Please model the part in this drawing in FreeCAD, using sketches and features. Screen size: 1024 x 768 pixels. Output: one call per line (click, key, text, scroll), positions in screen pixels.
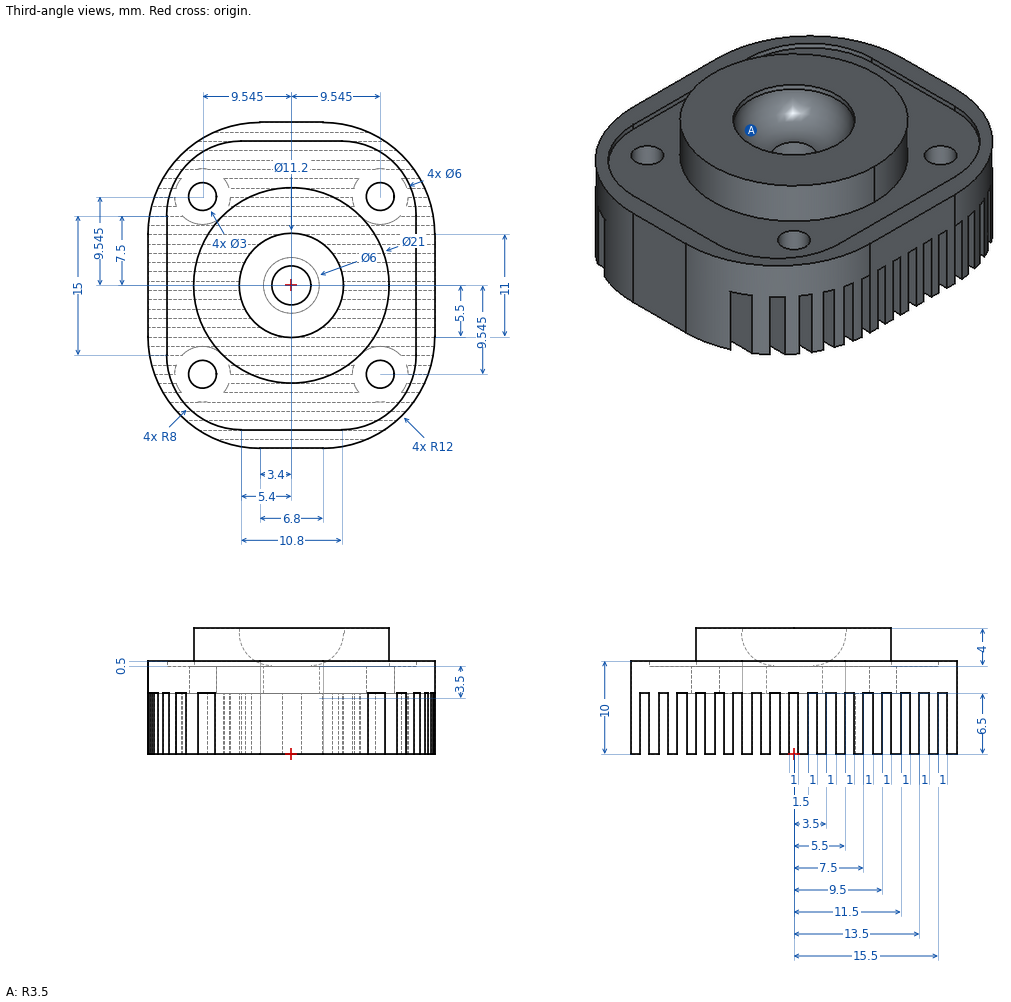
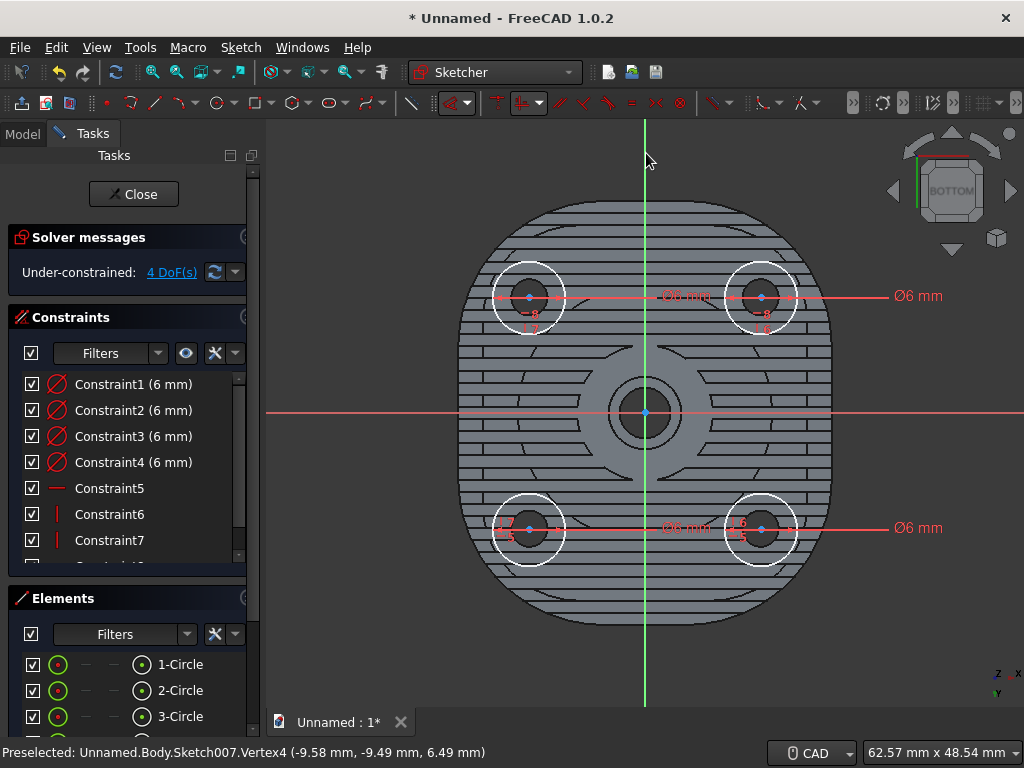
click(761, 530)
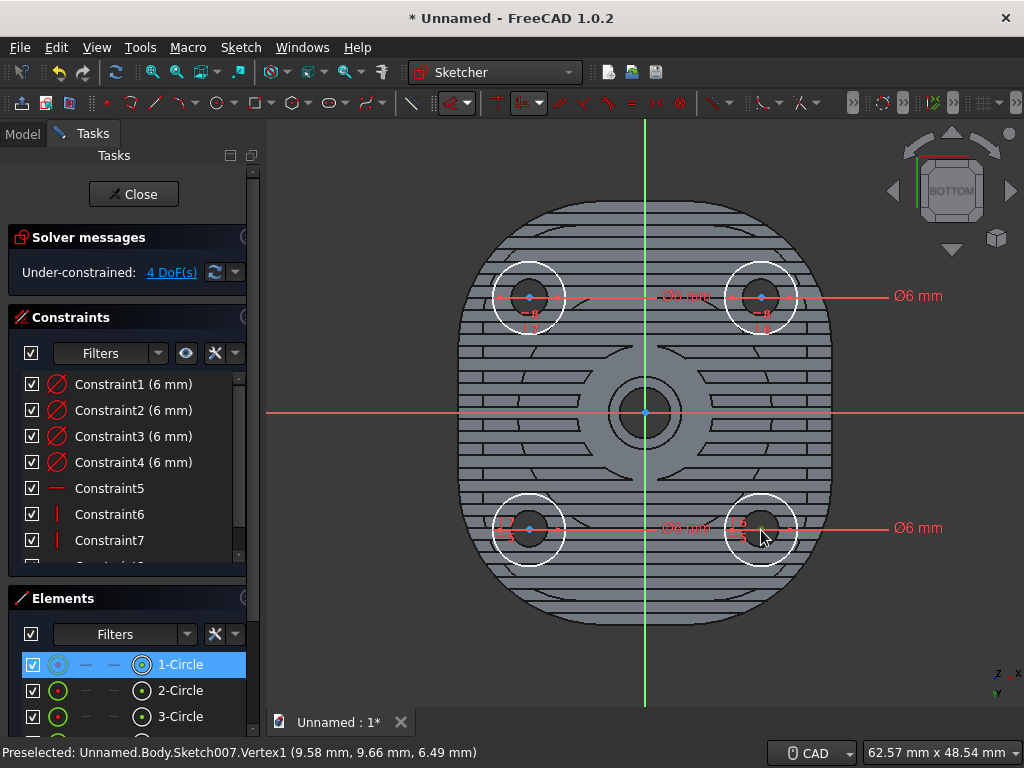
key(l)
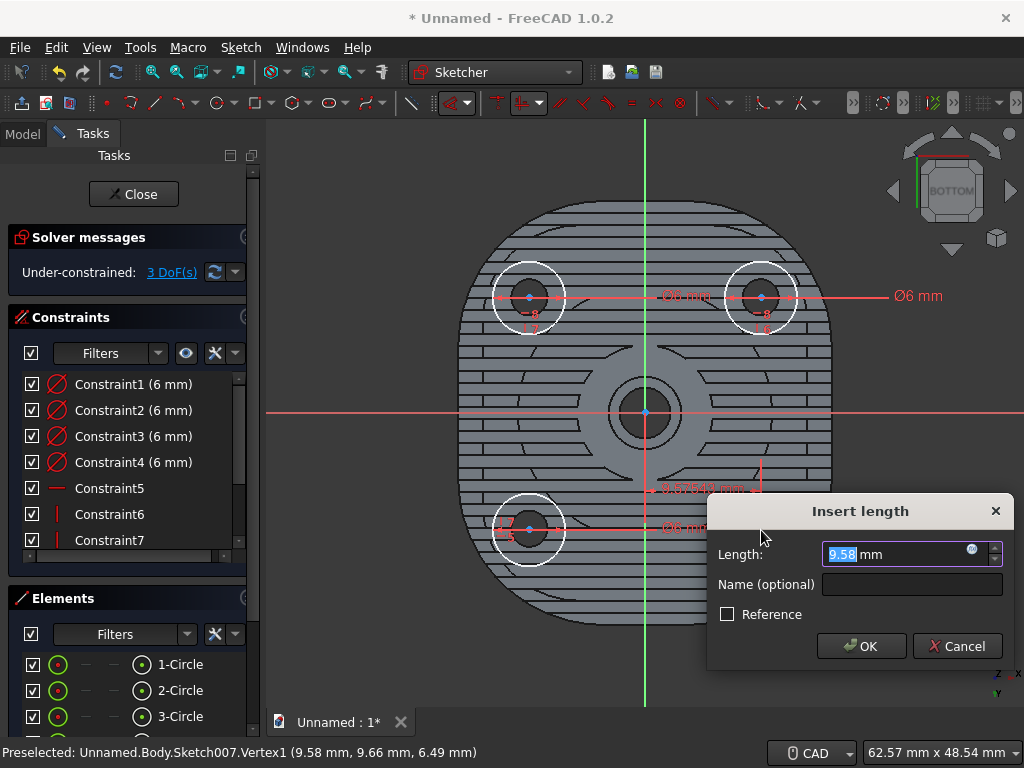
text(9.545)
key(Return)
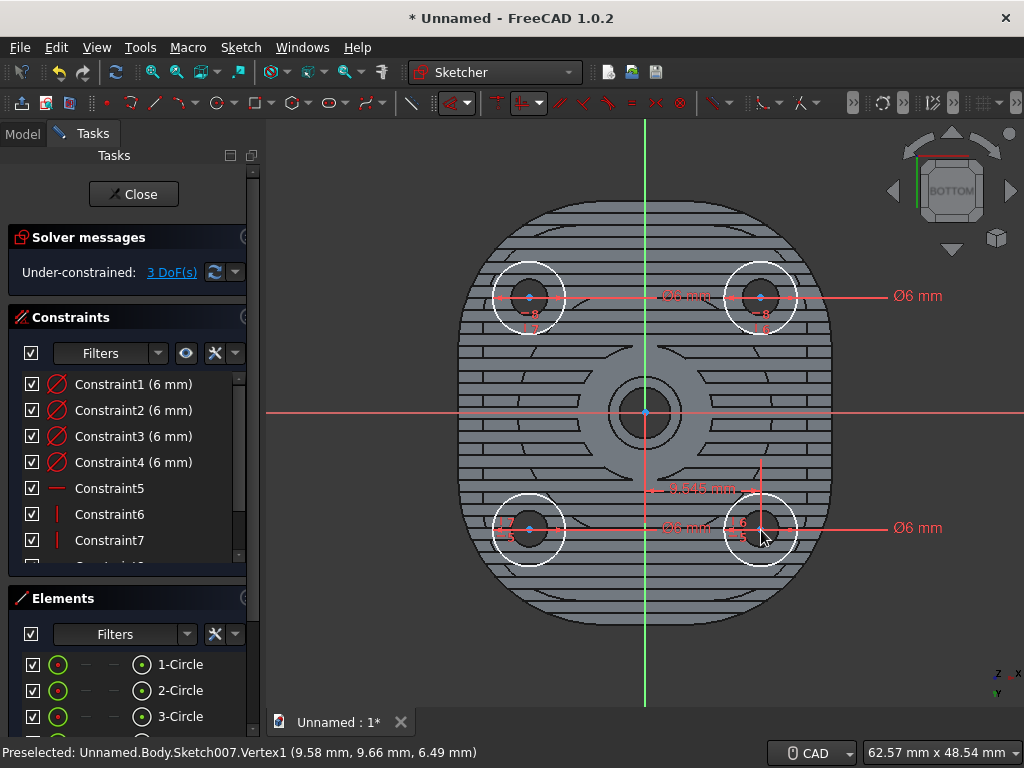
click(761, 530)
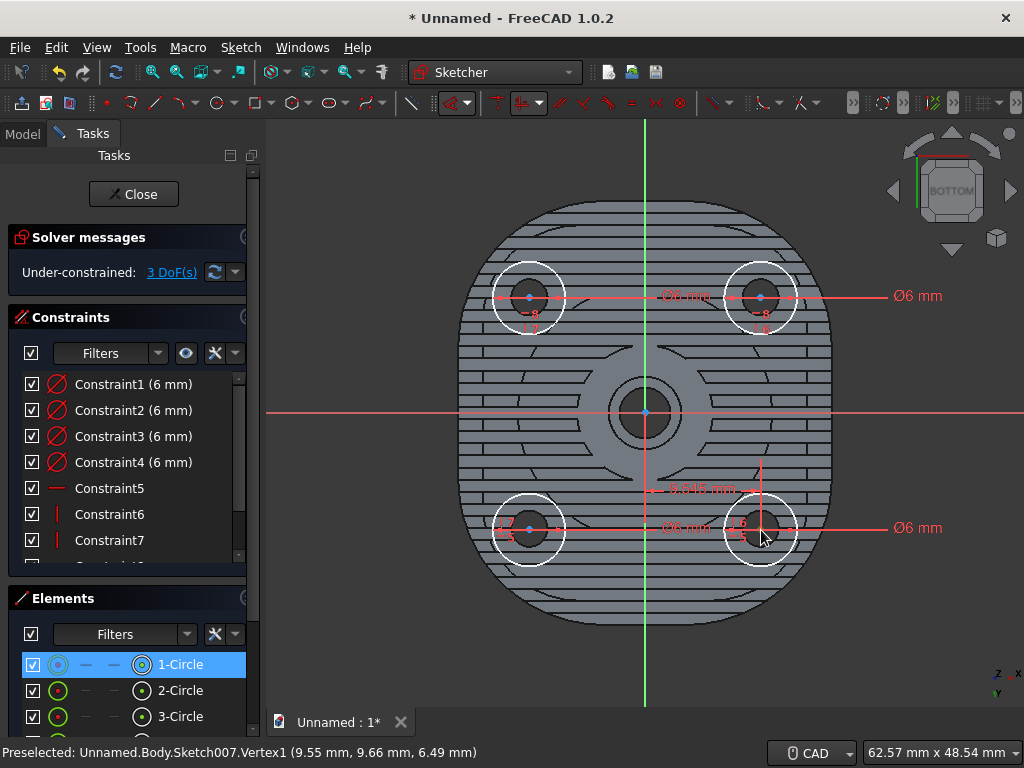
key(i)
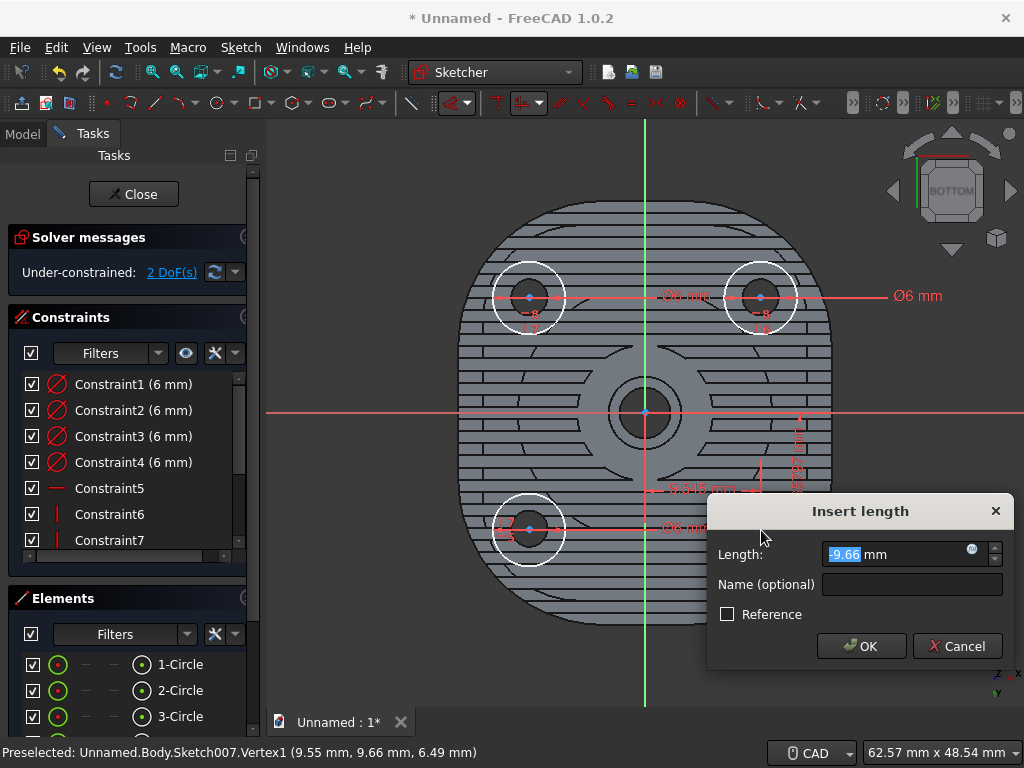
text(-9.545)
key(Return)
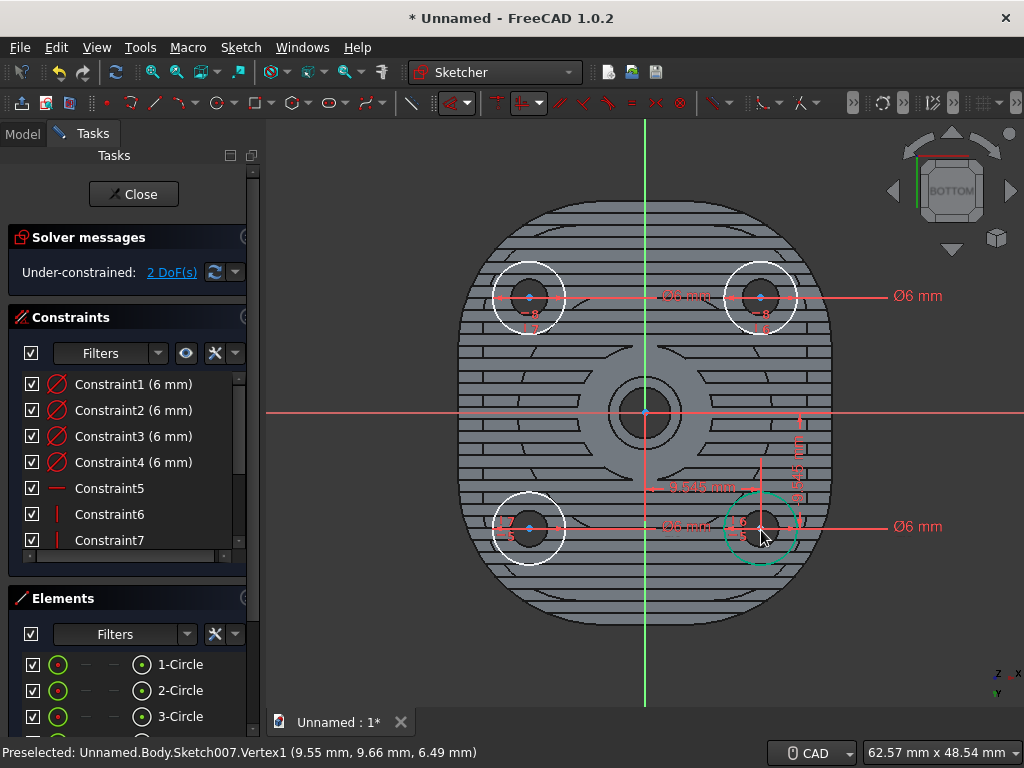
click(529, 529)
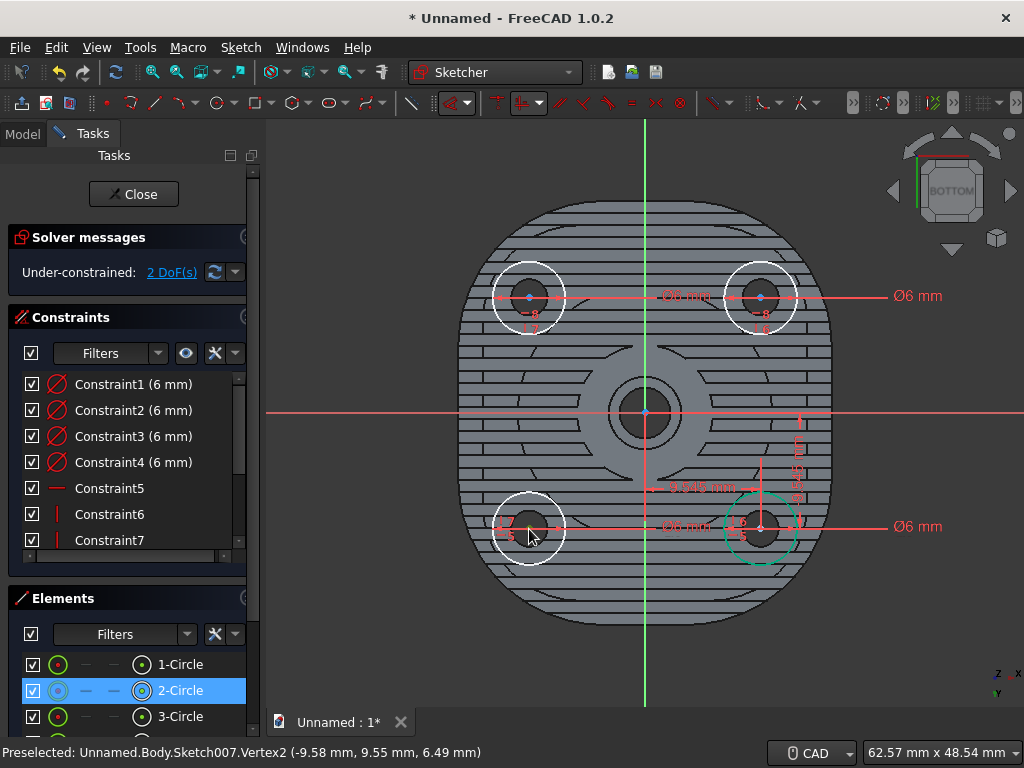
key(l)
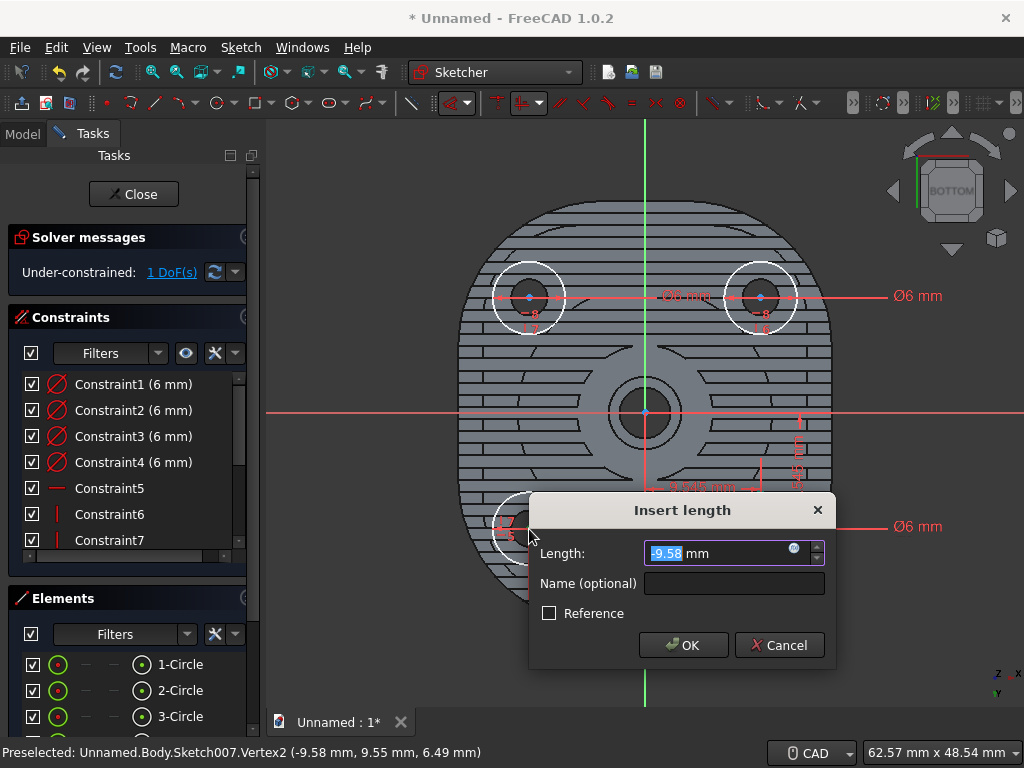
text(-9.545)
key(Return)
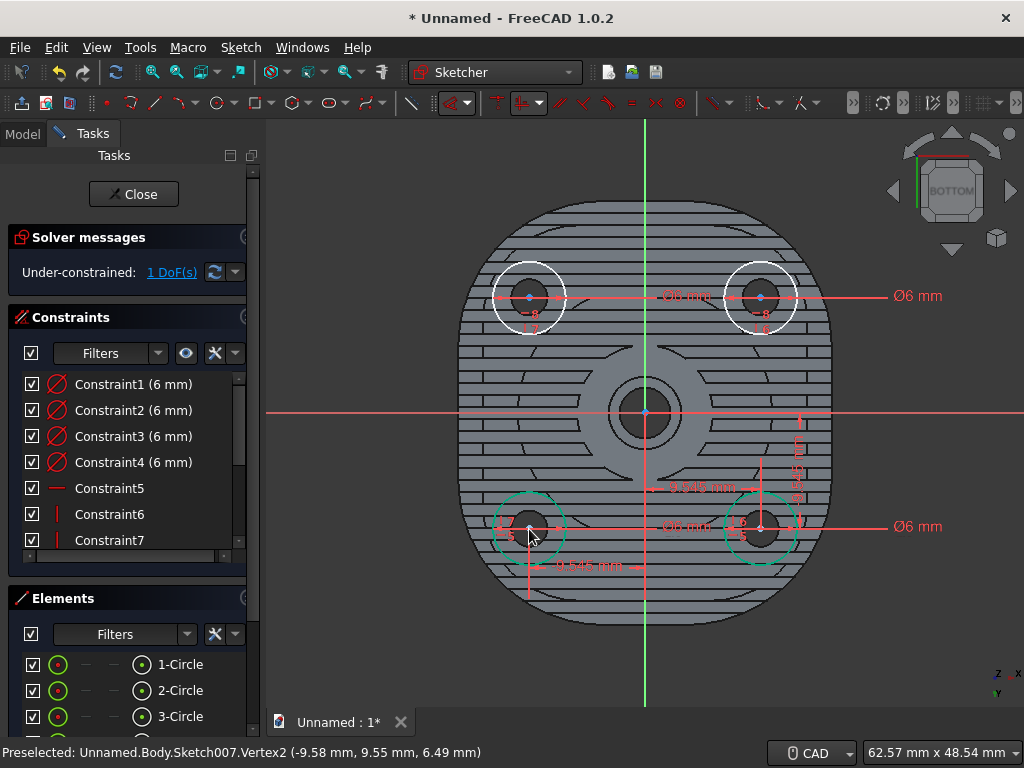
click(761, 298)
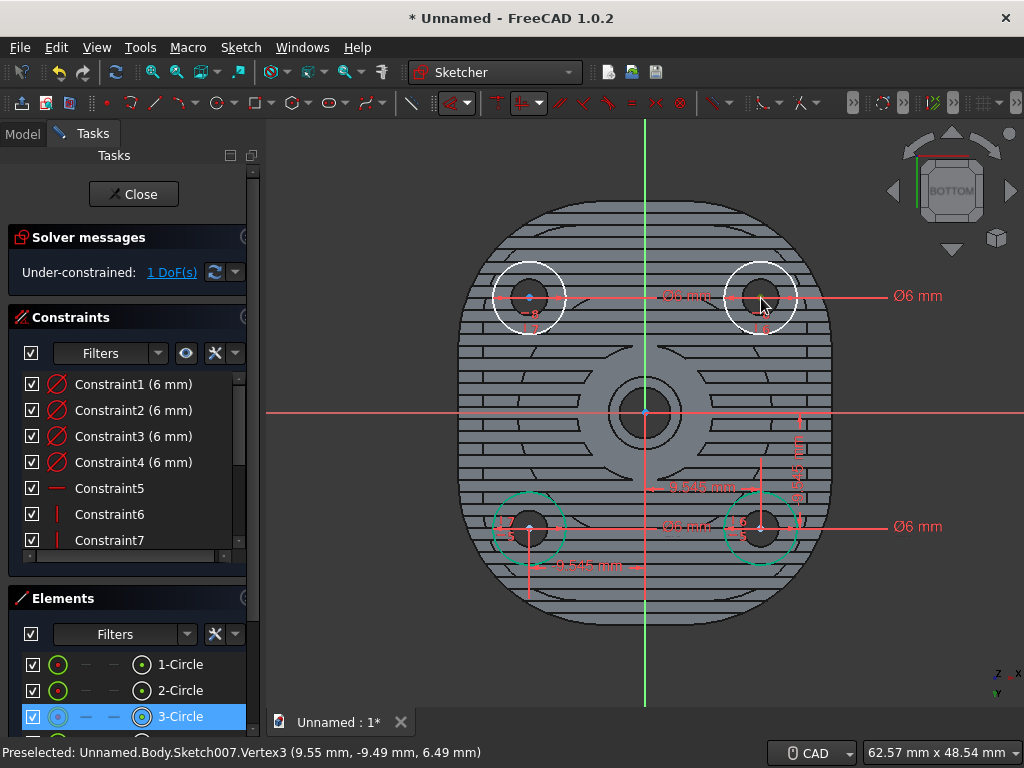
key(i)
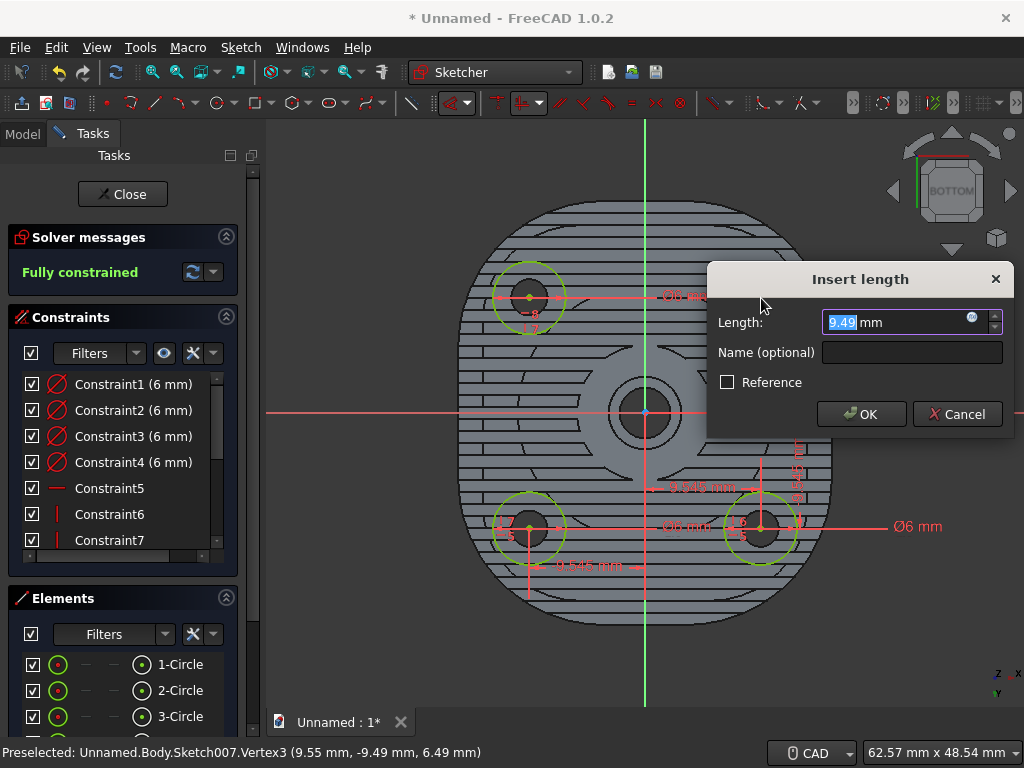
text(9.545)
key(Return)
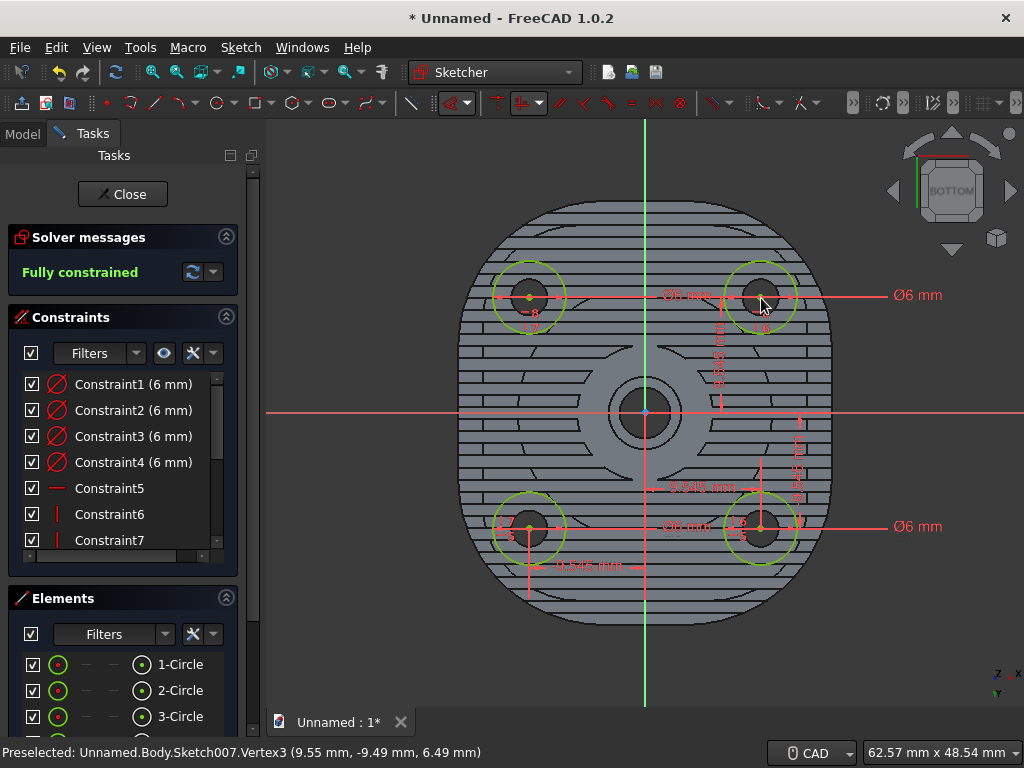
click(123, 194)